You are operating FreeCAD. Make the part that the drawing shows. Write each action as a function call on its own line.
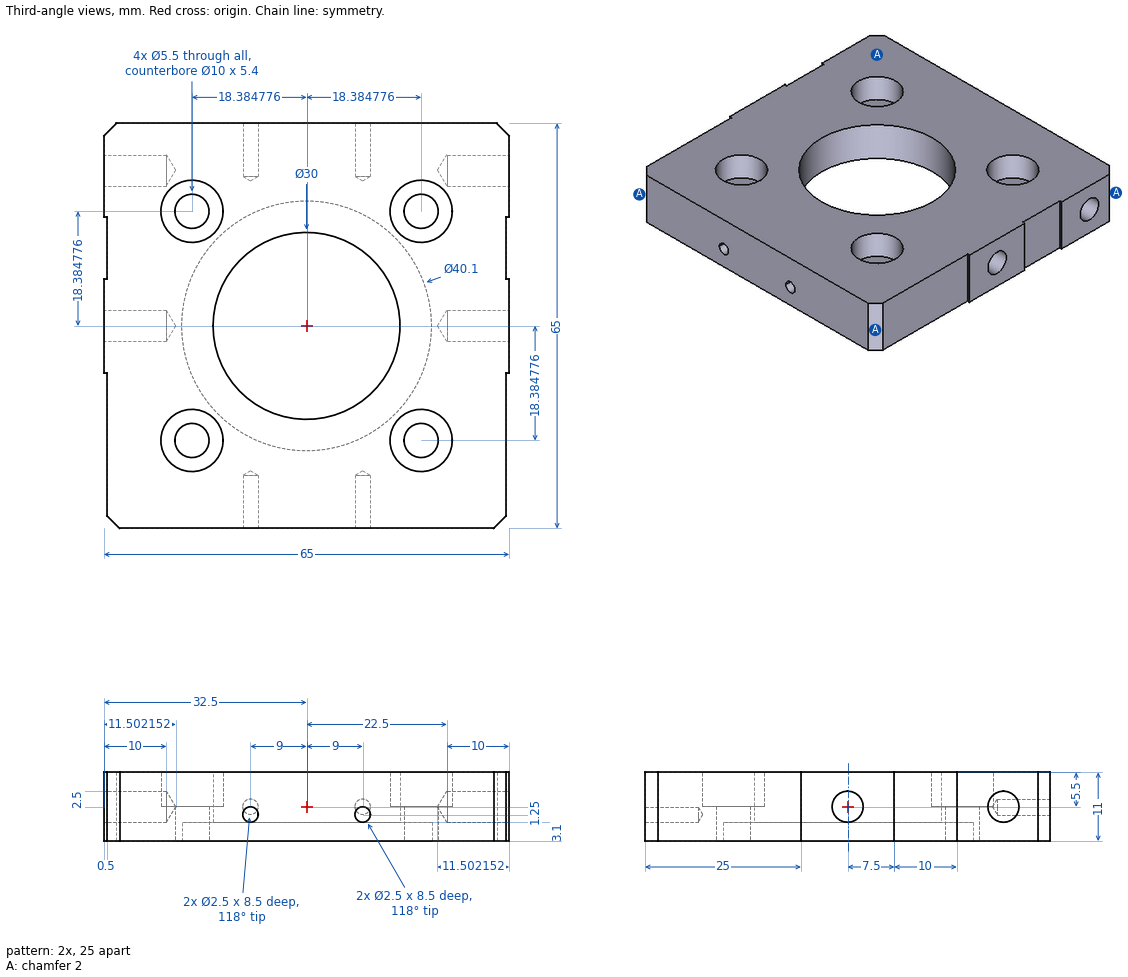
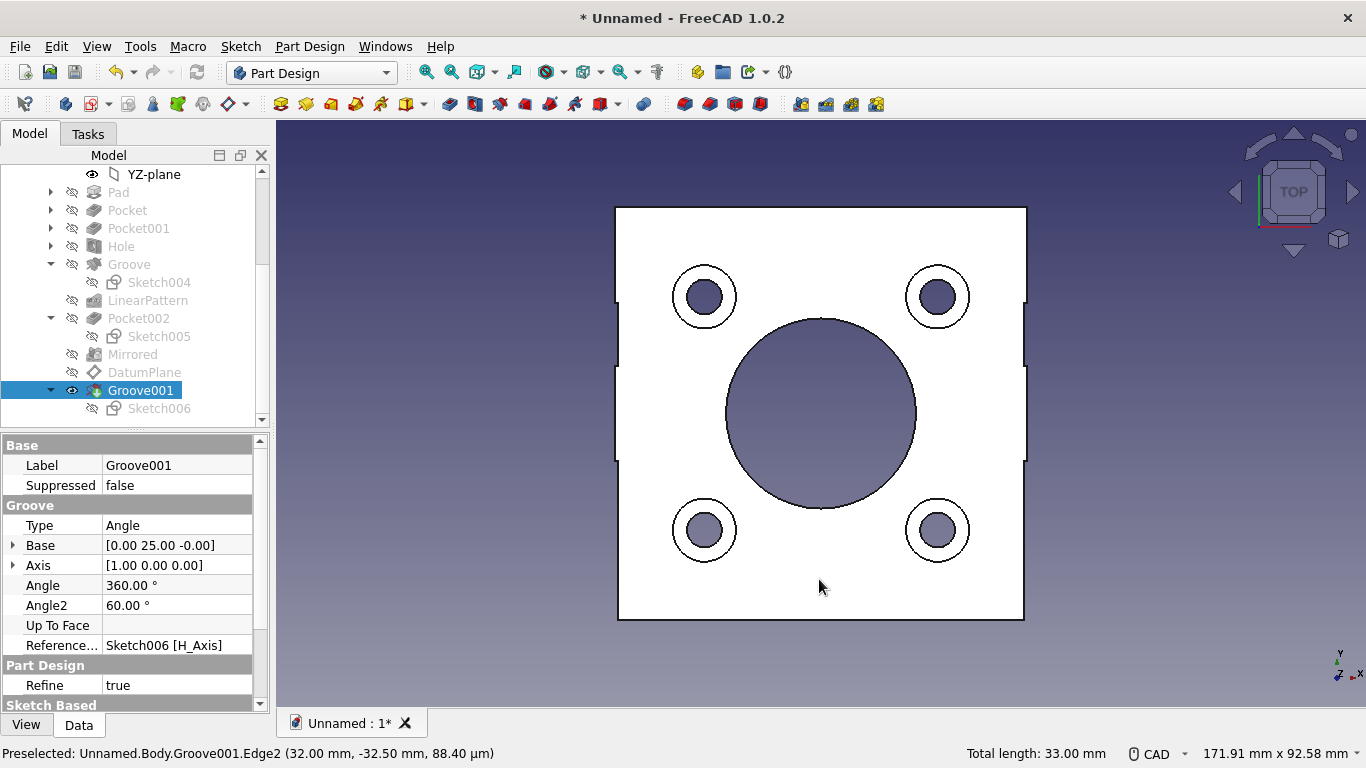
key(1)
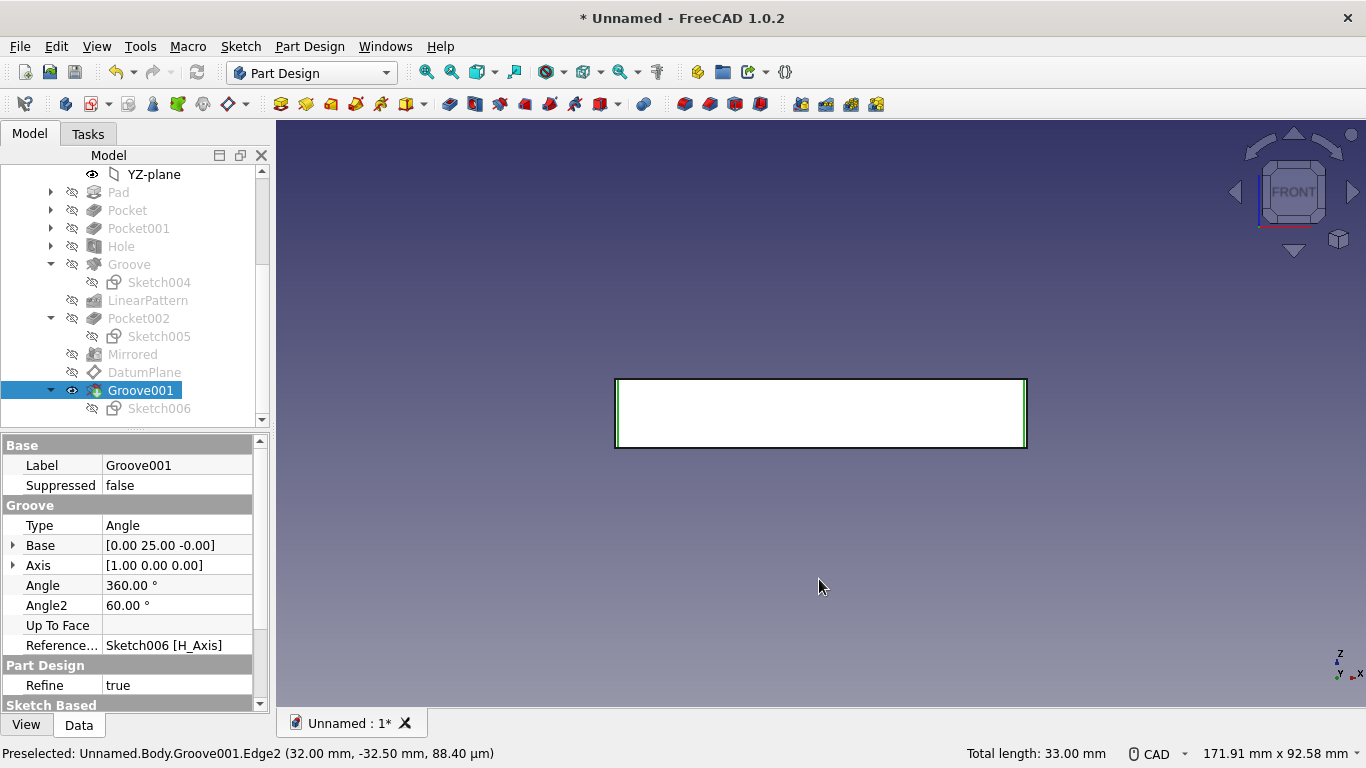
click(427, 72)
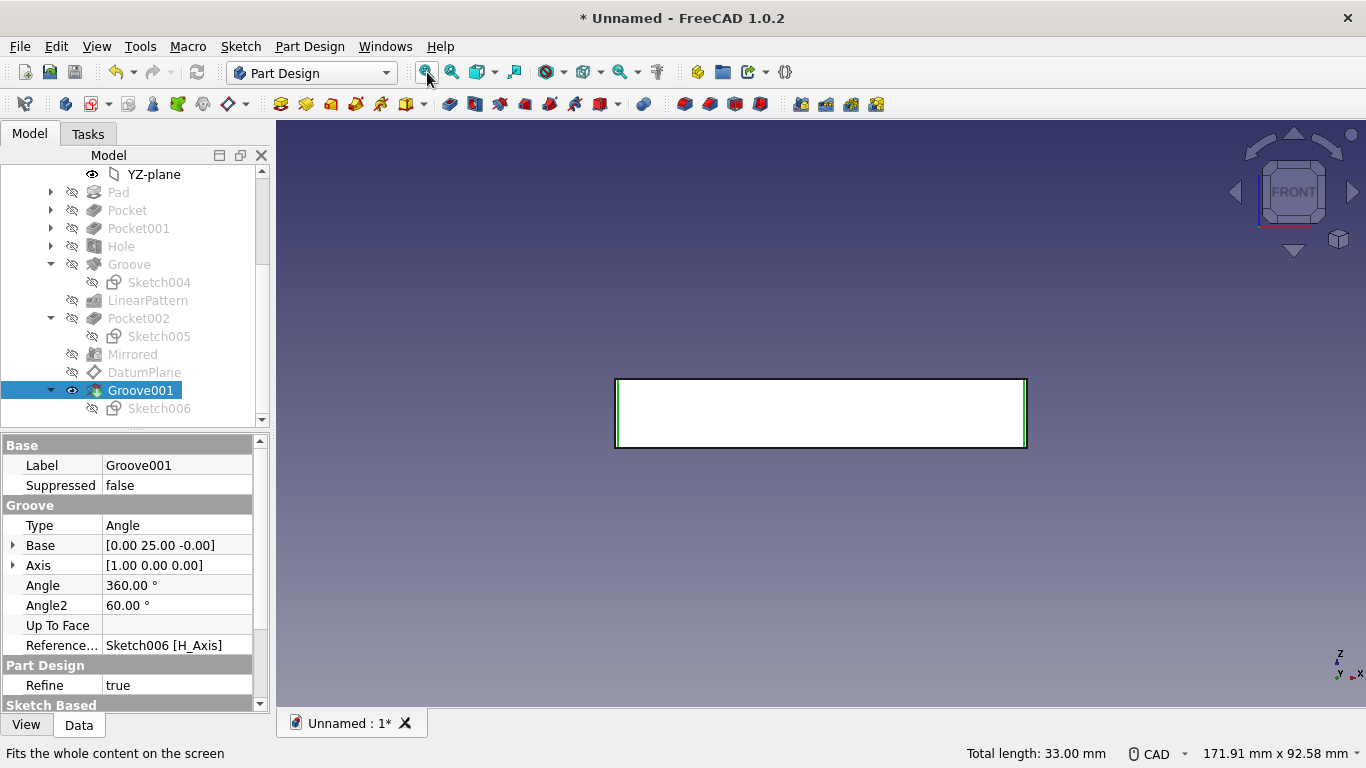
key(3)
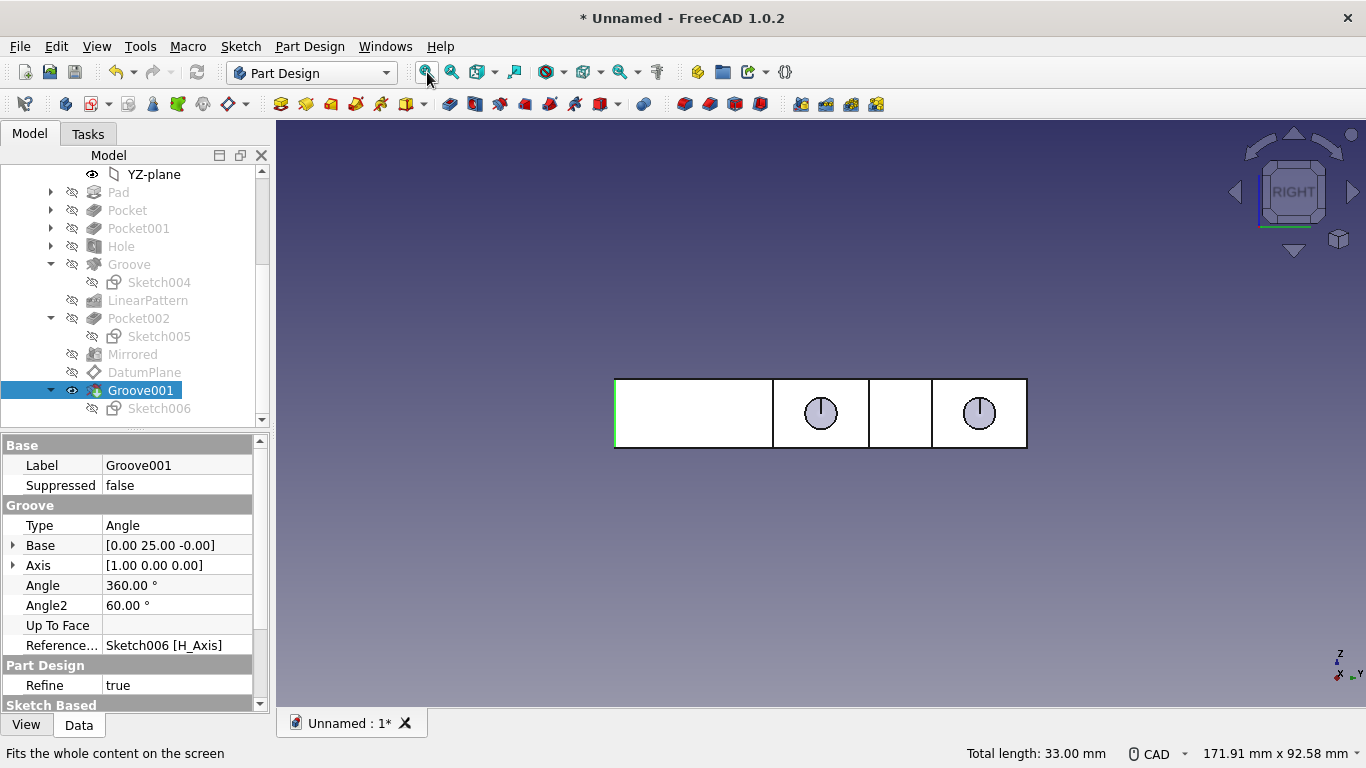
click(427, 72)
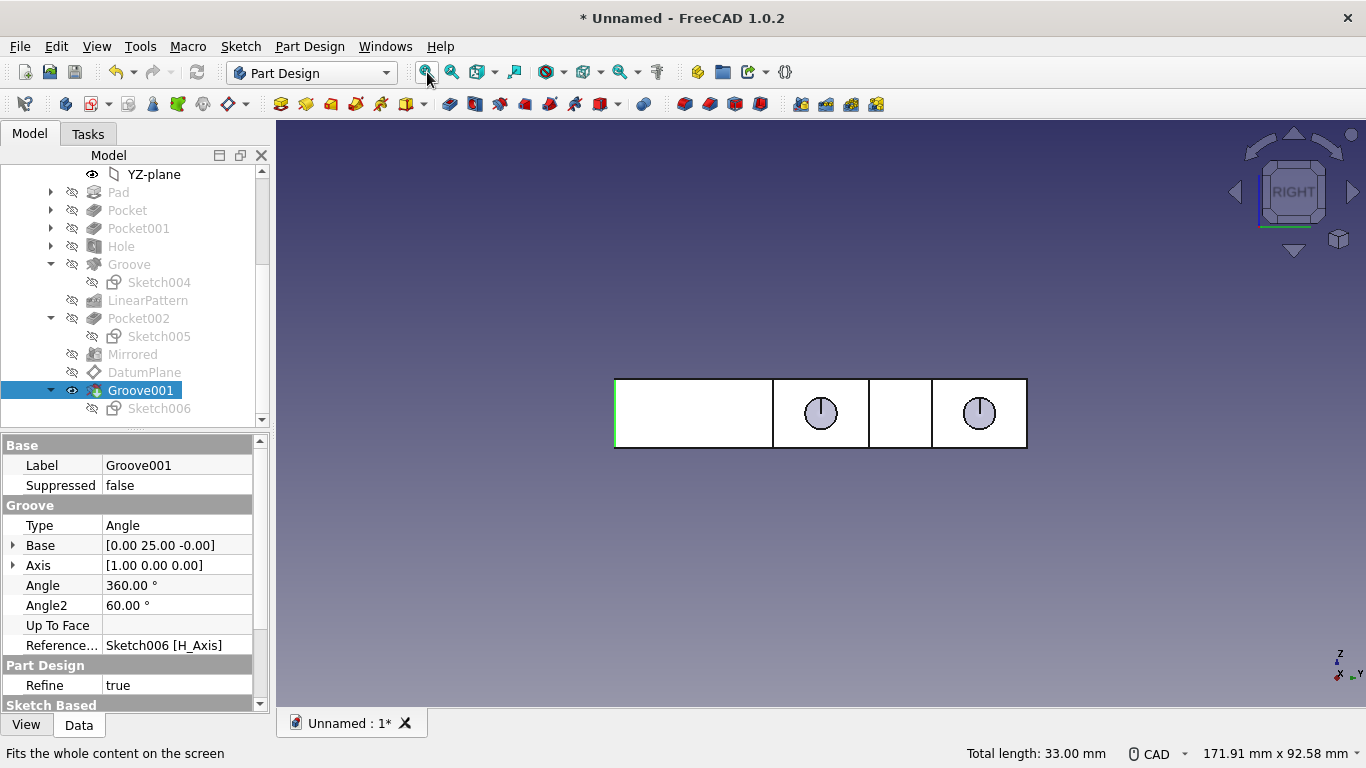
click(1027, 412, ctrl)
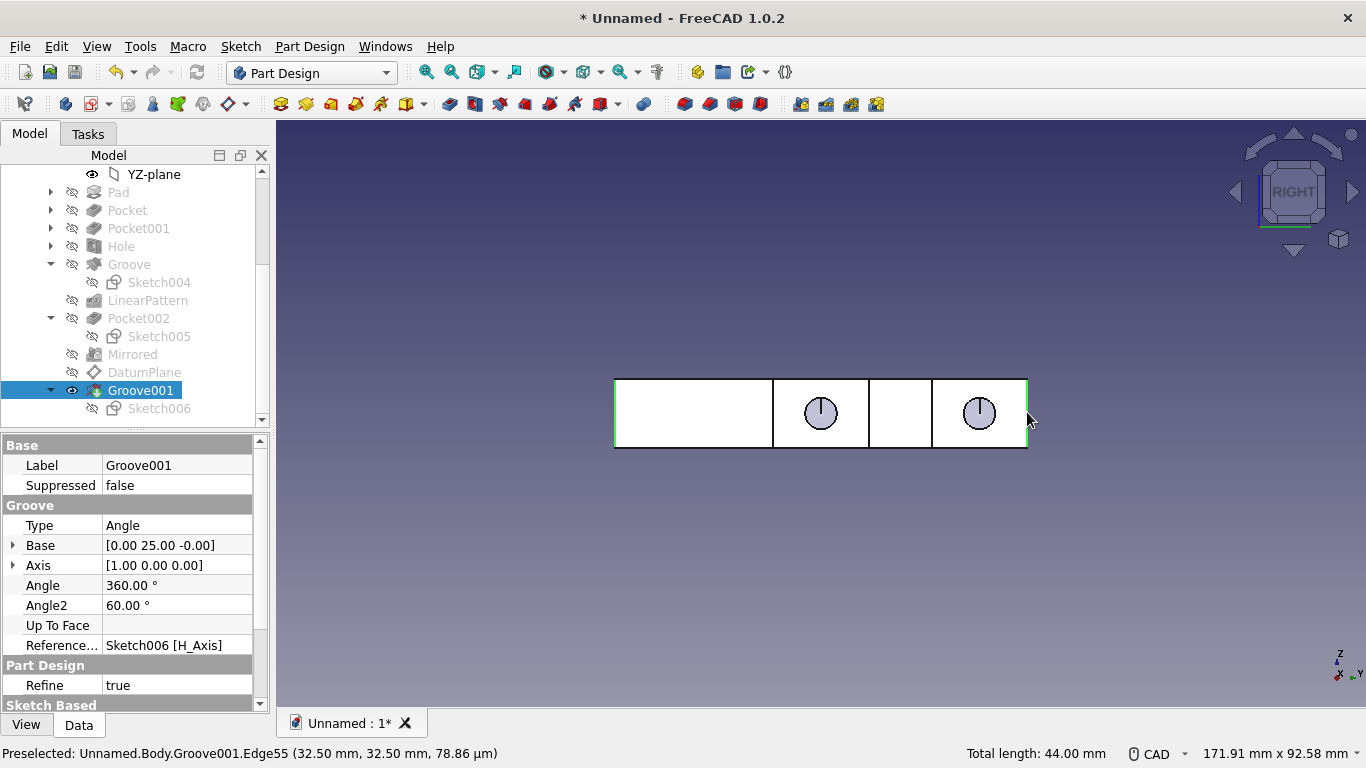
click(710, 104)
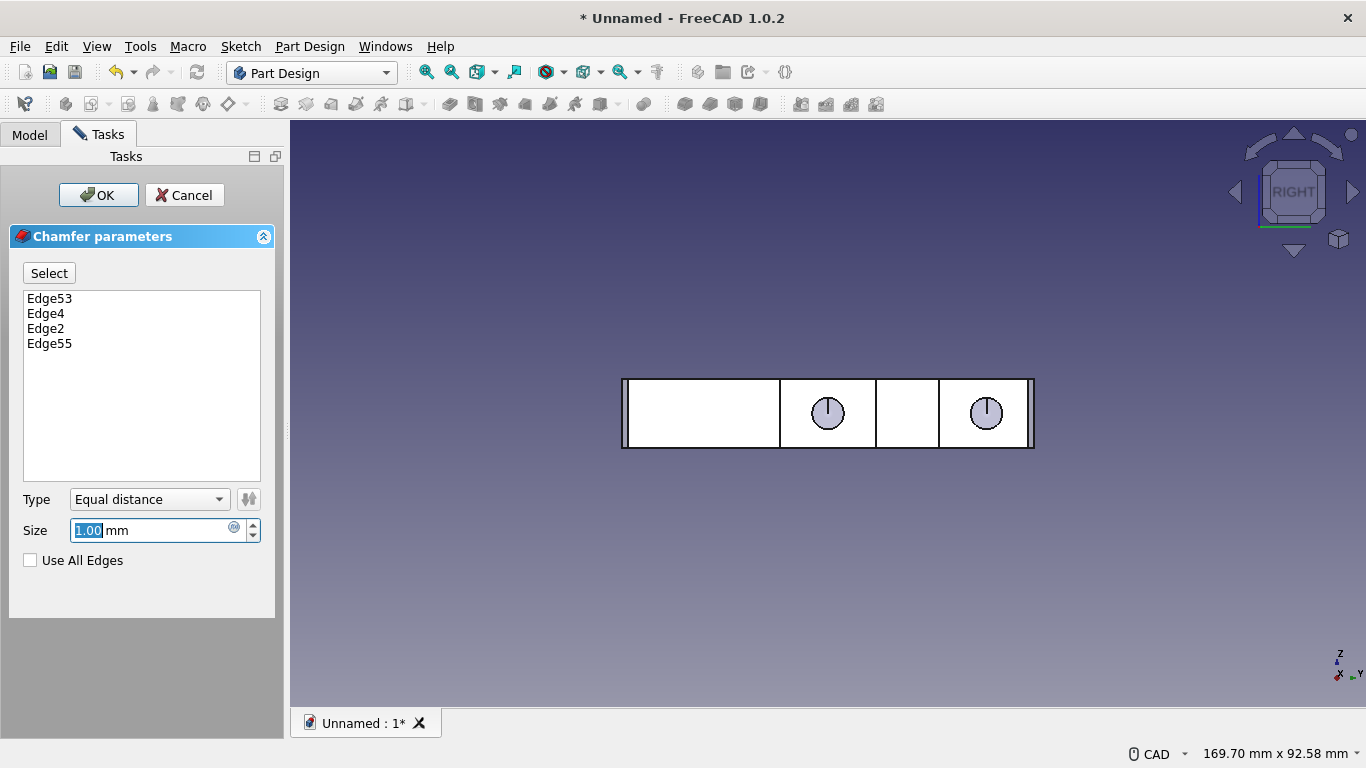
text(2)
key(Tab)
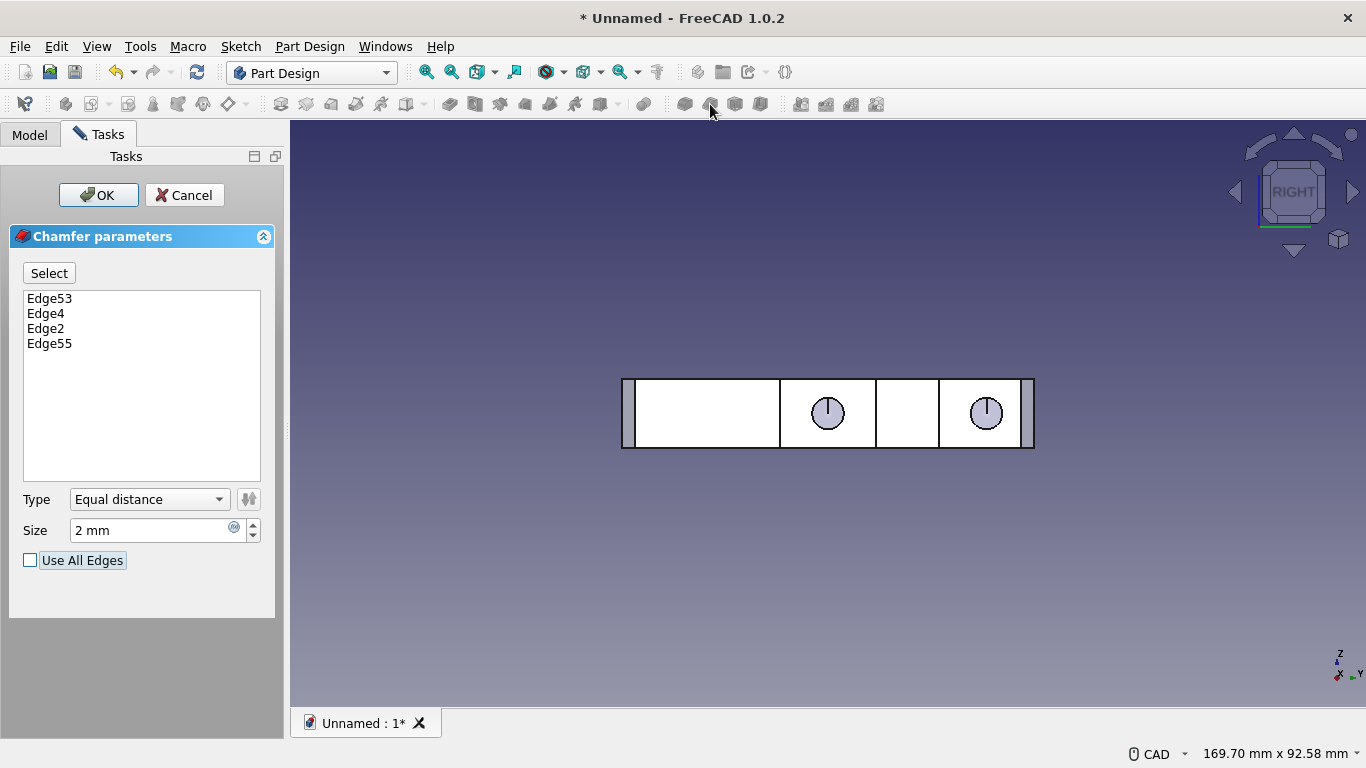
click(99, 195)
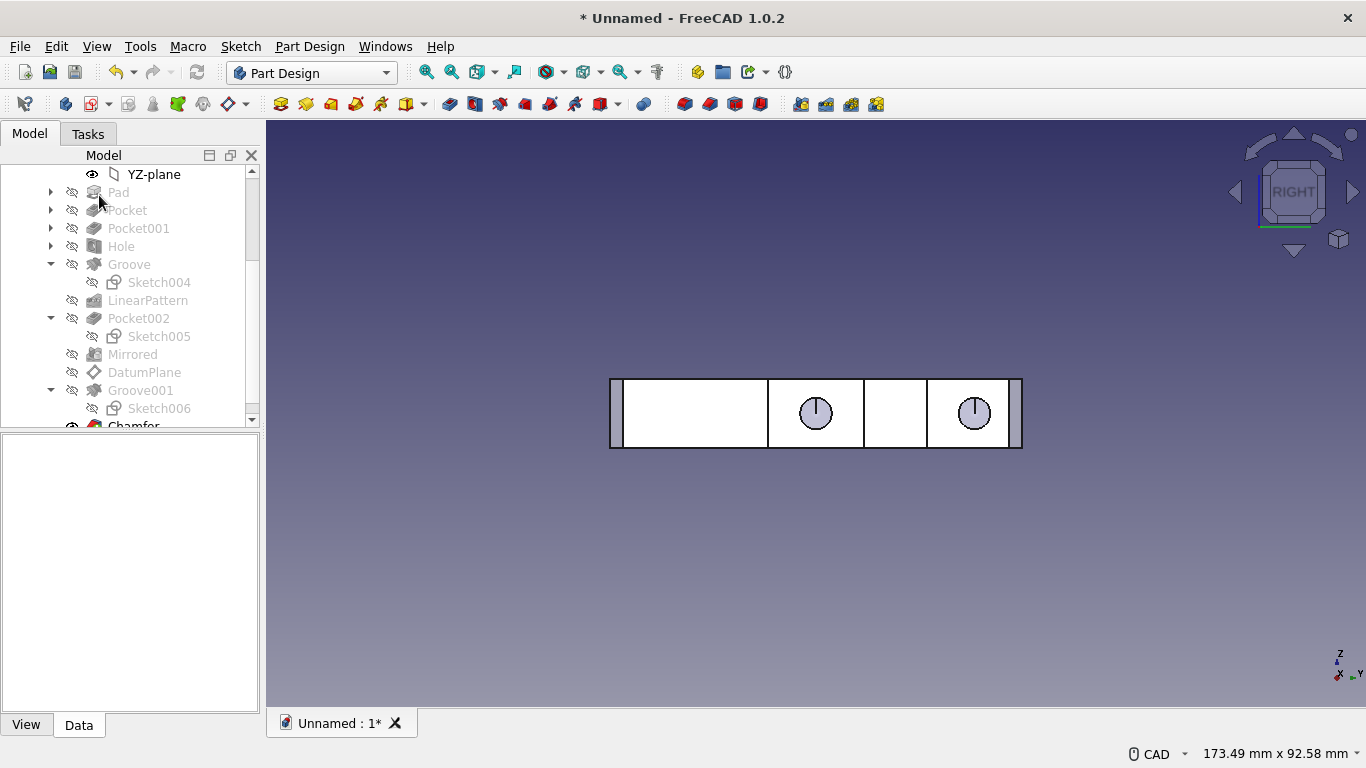
click(427, 72)